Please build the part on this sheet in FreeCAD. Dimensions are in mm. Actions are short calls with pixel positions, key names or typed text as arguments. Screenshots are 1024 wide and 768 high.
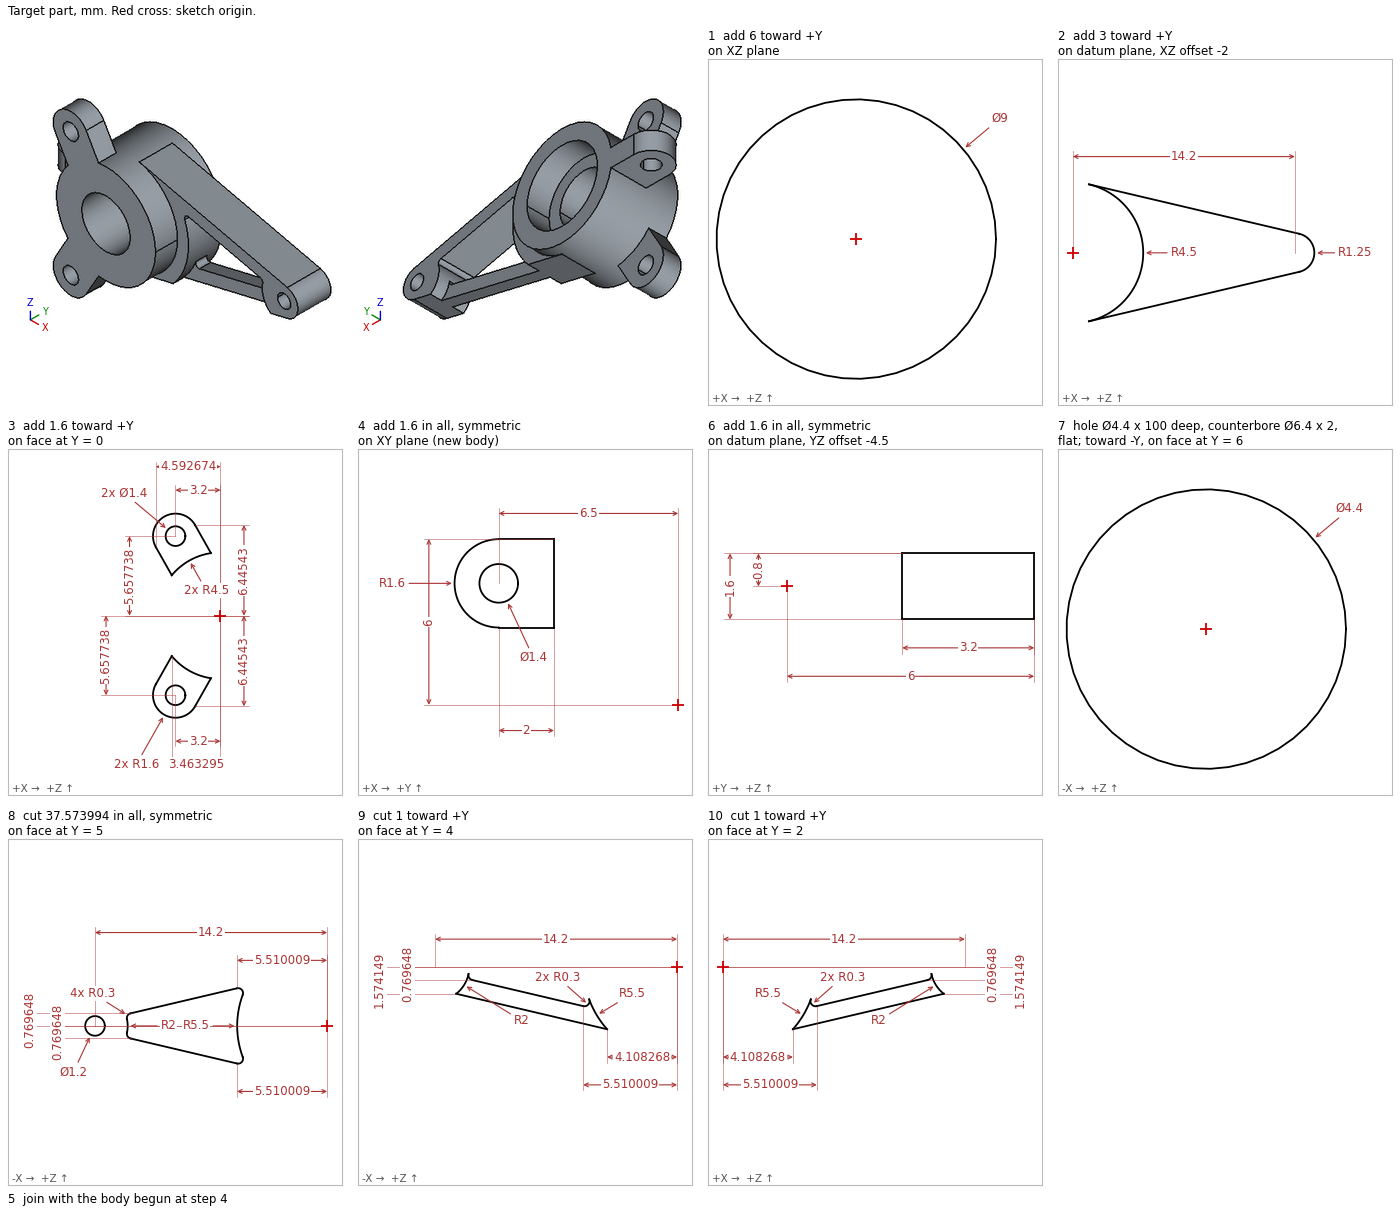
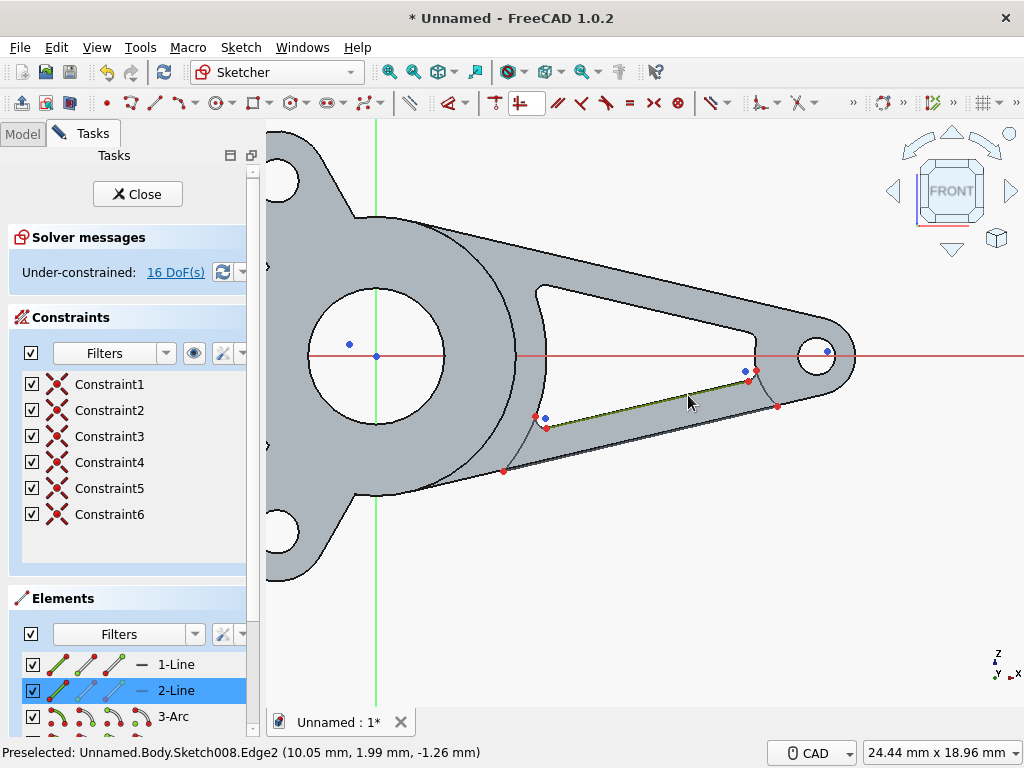
scroll(541, 427, up, 5)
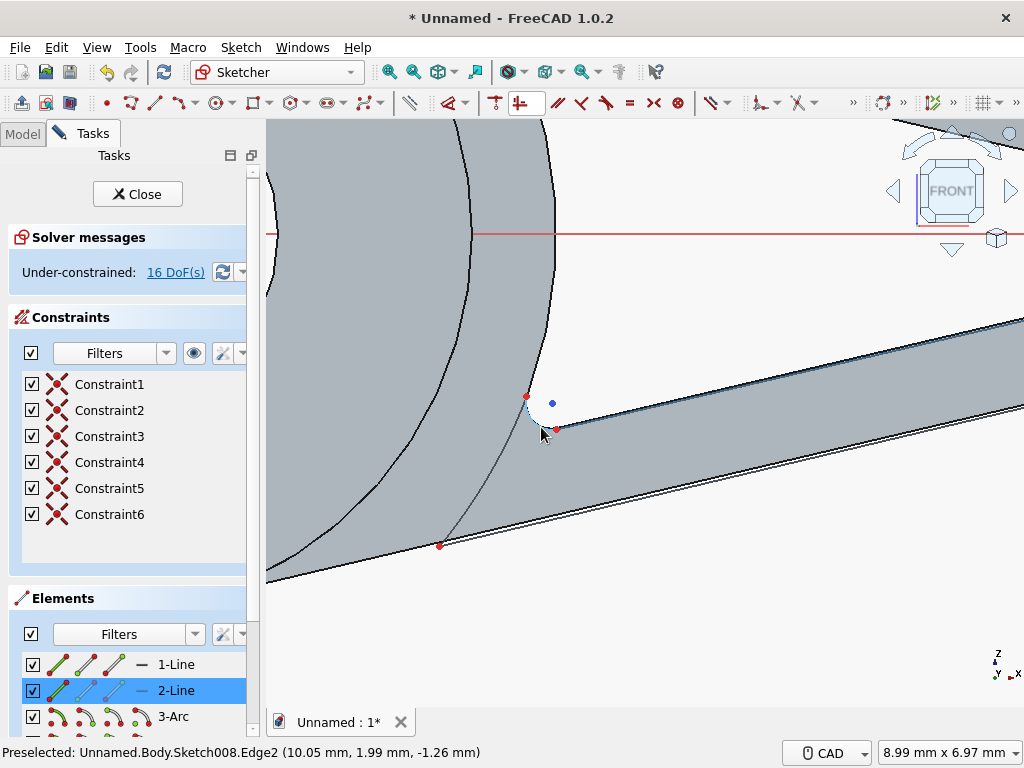
click(541, 427)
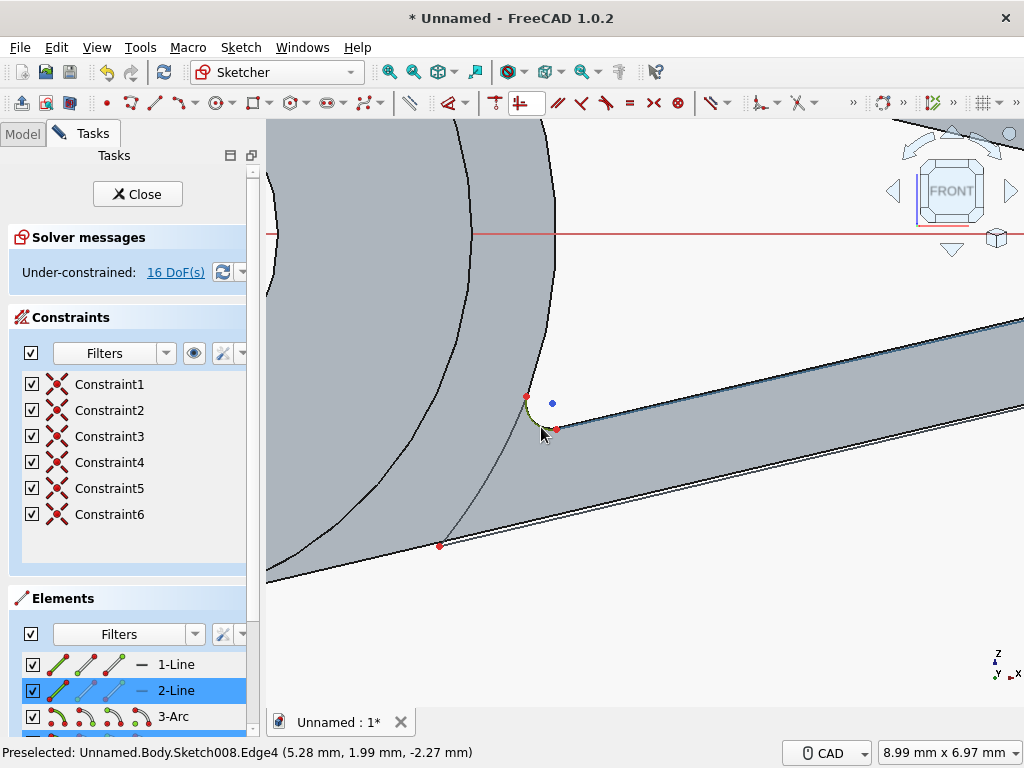
click(606, 104)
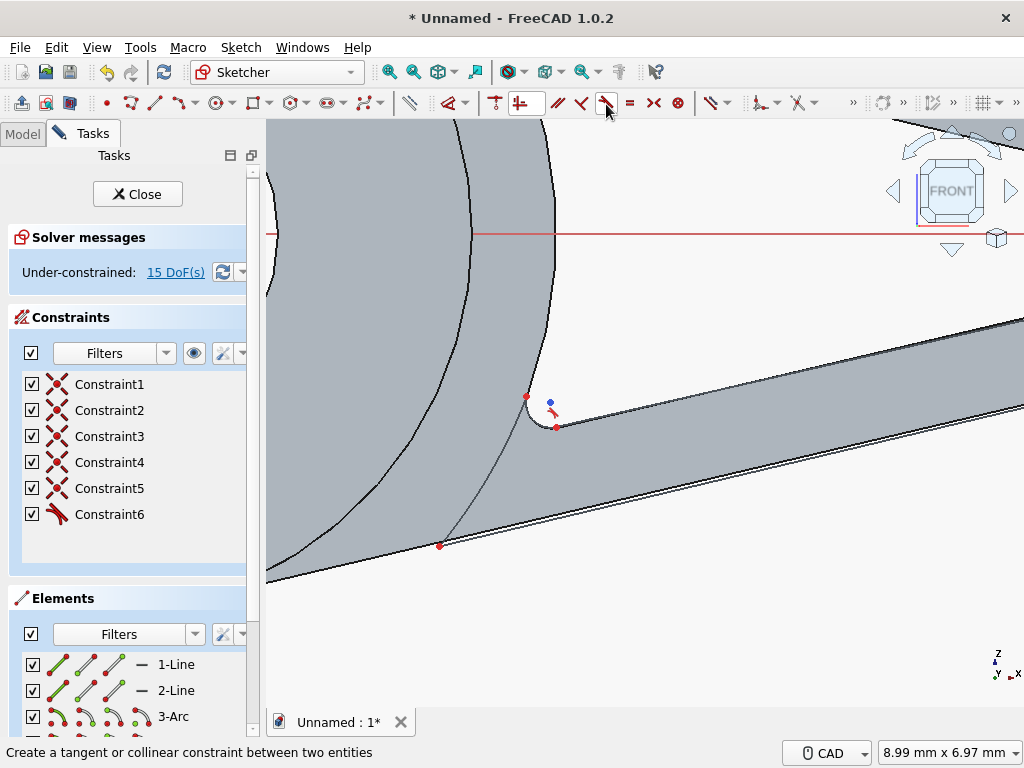
click(721, 389)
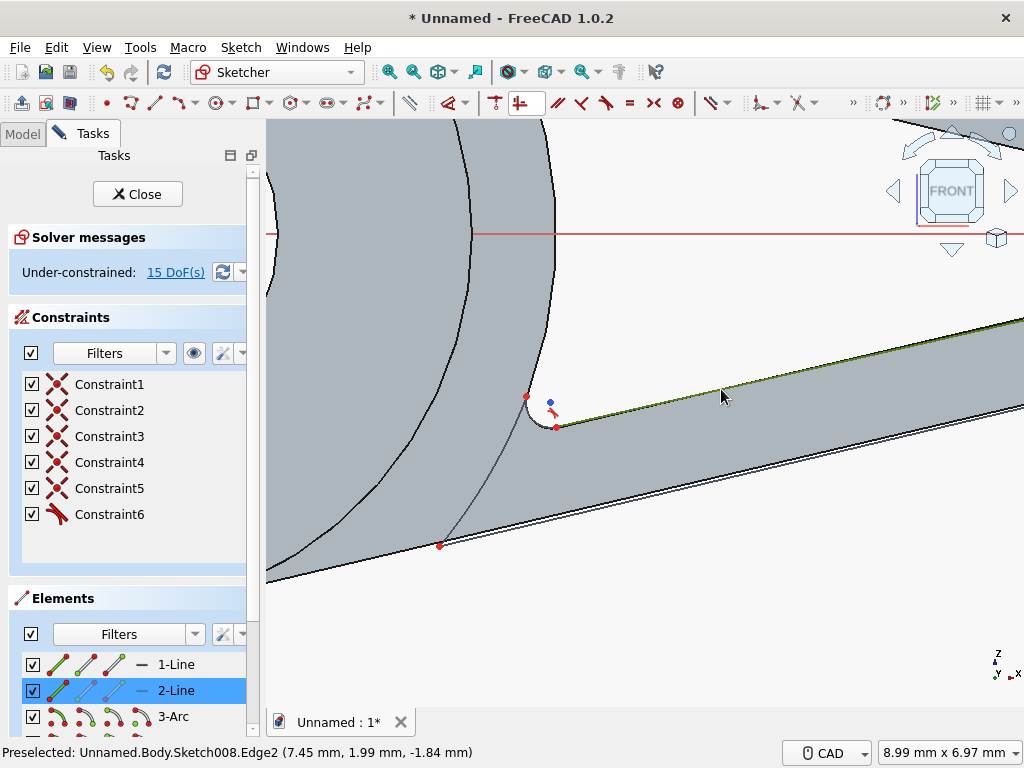
scroll(540, 427, down, 5)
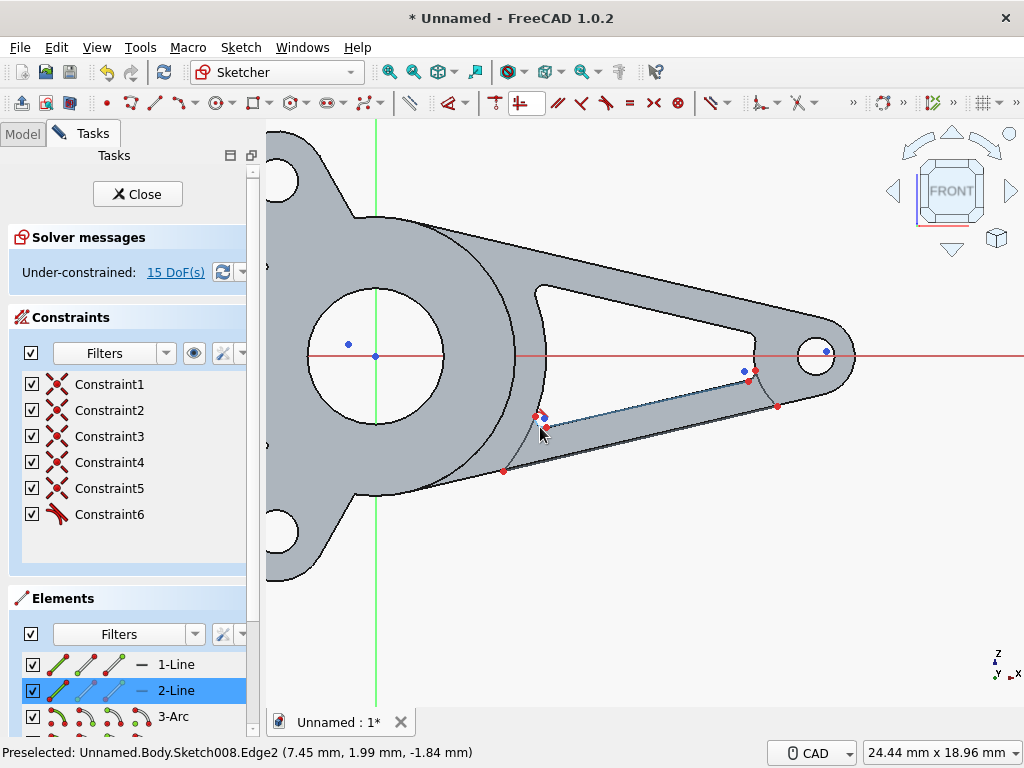
scroll(752, 379, up, 6)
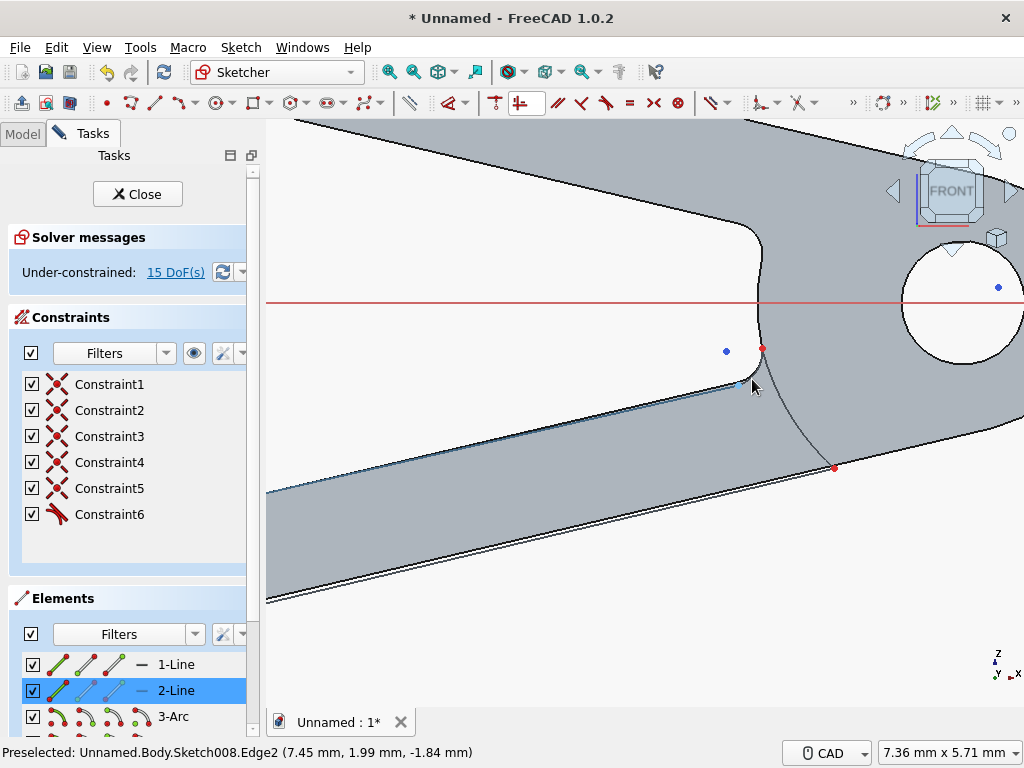
click(750, 378)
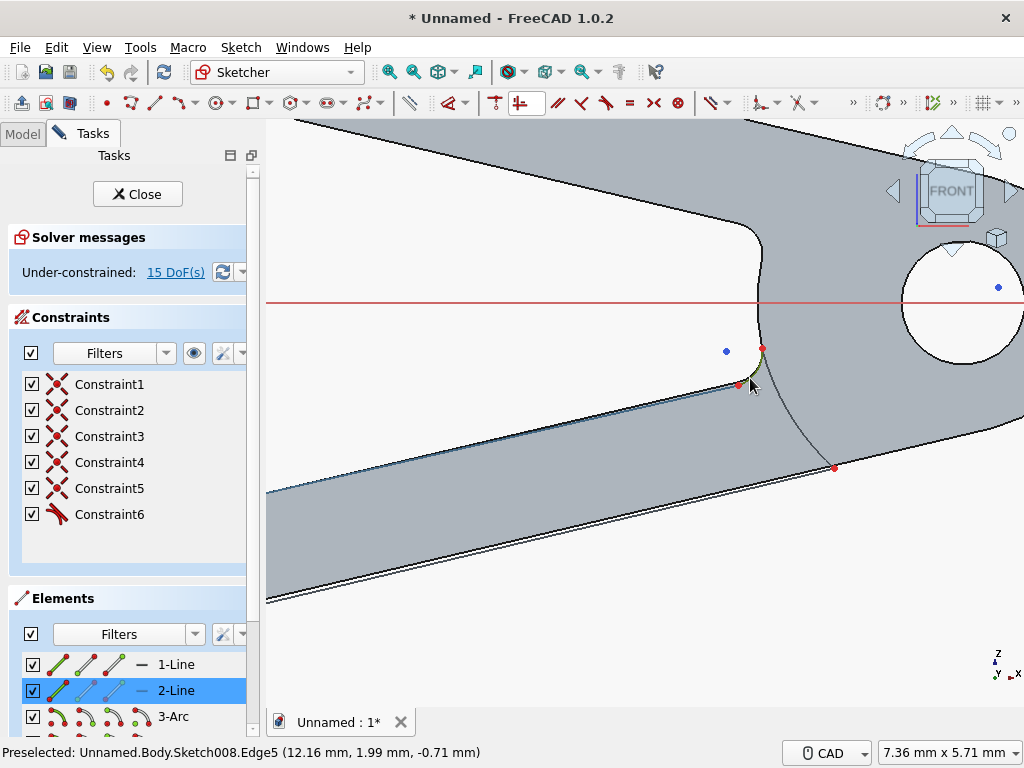
key(t)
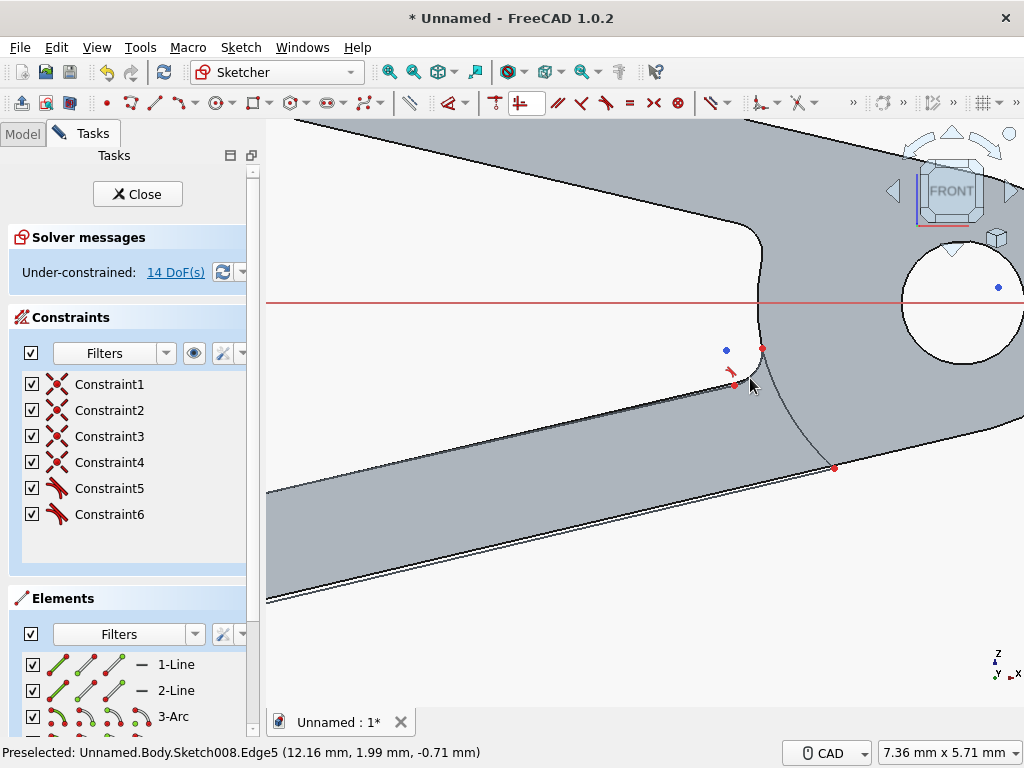
scroll(752, 379, down, 6)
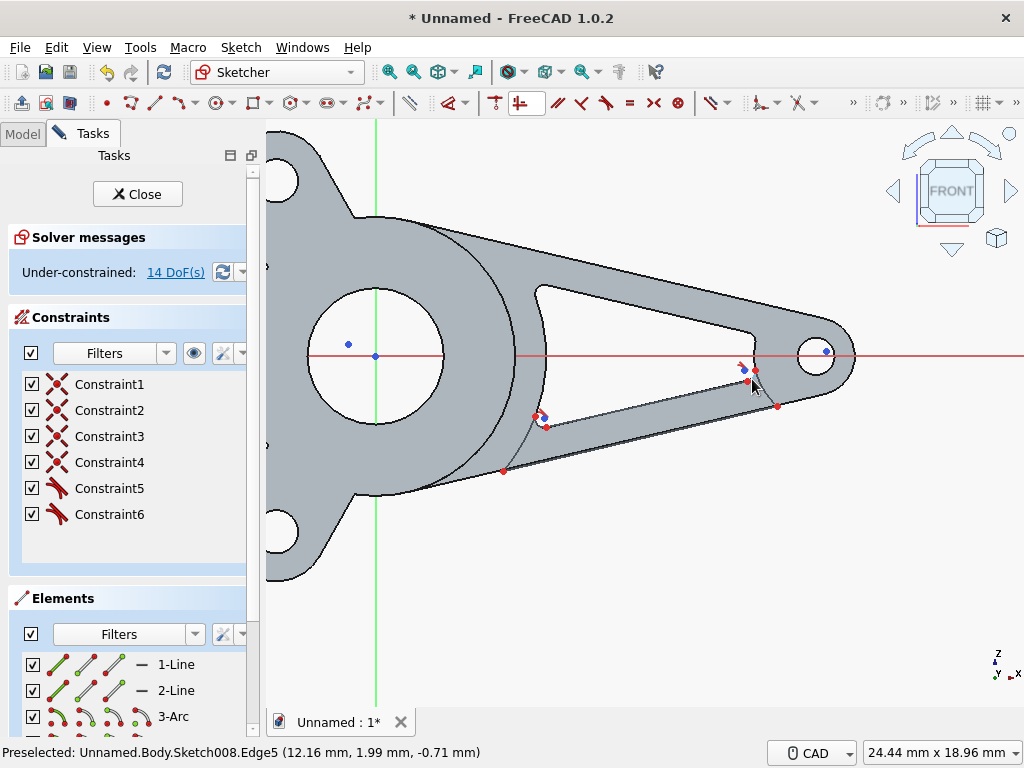
click(515, 456)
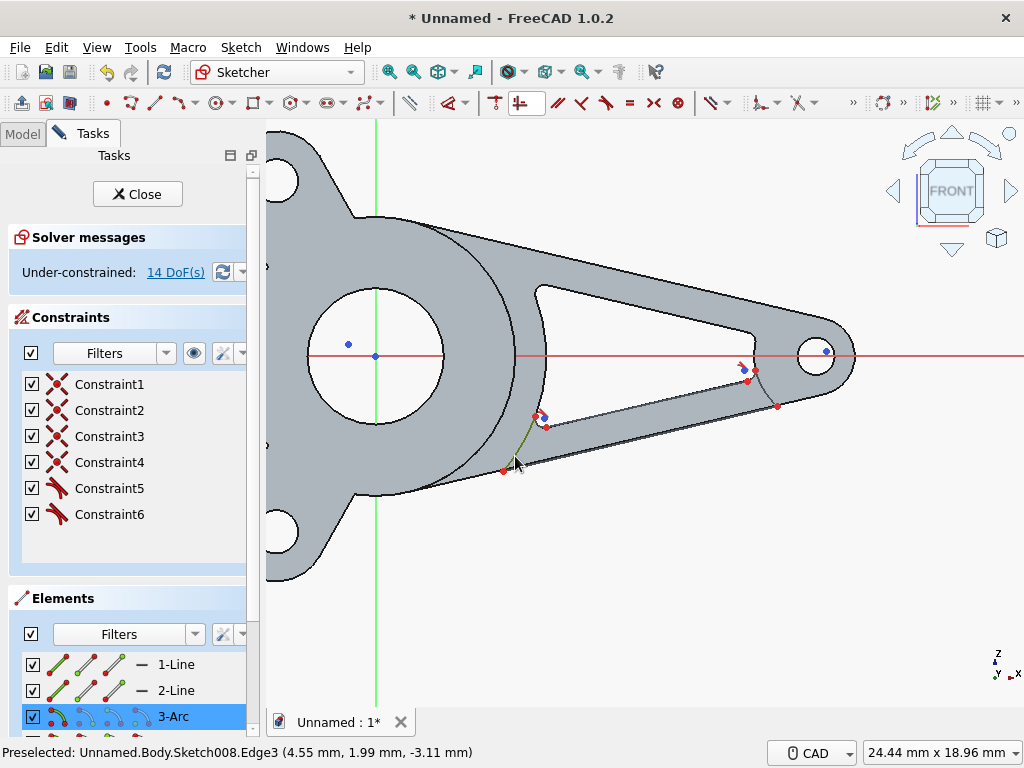
scroll(541, 427, up, 5)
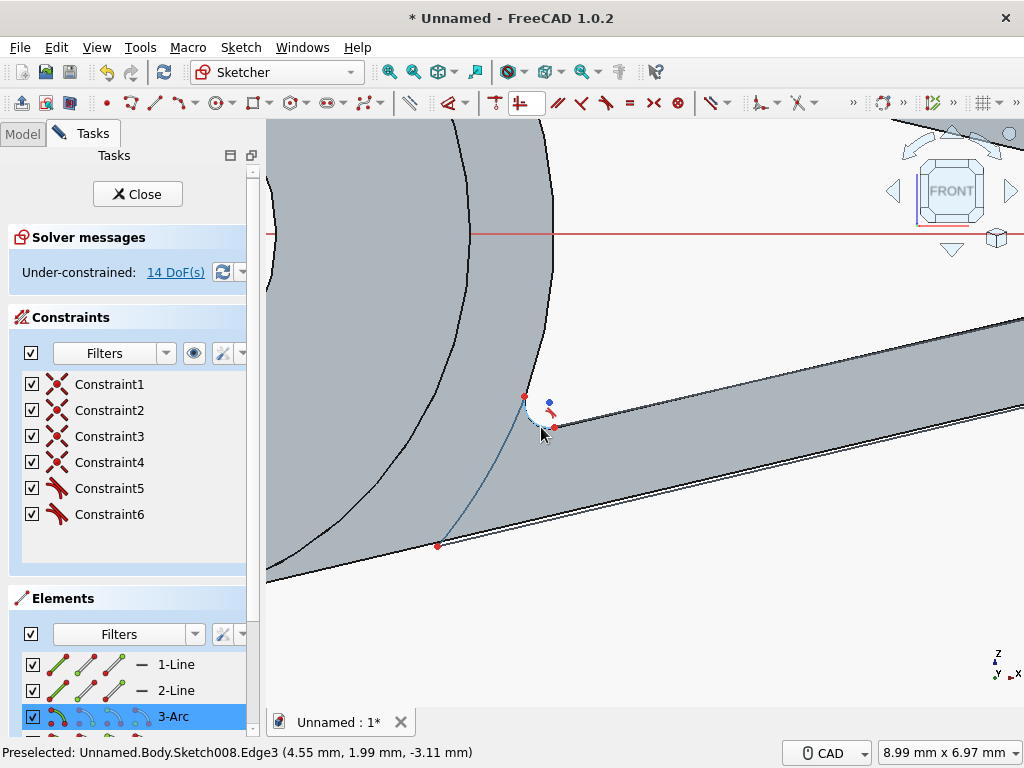
click(540, 426)